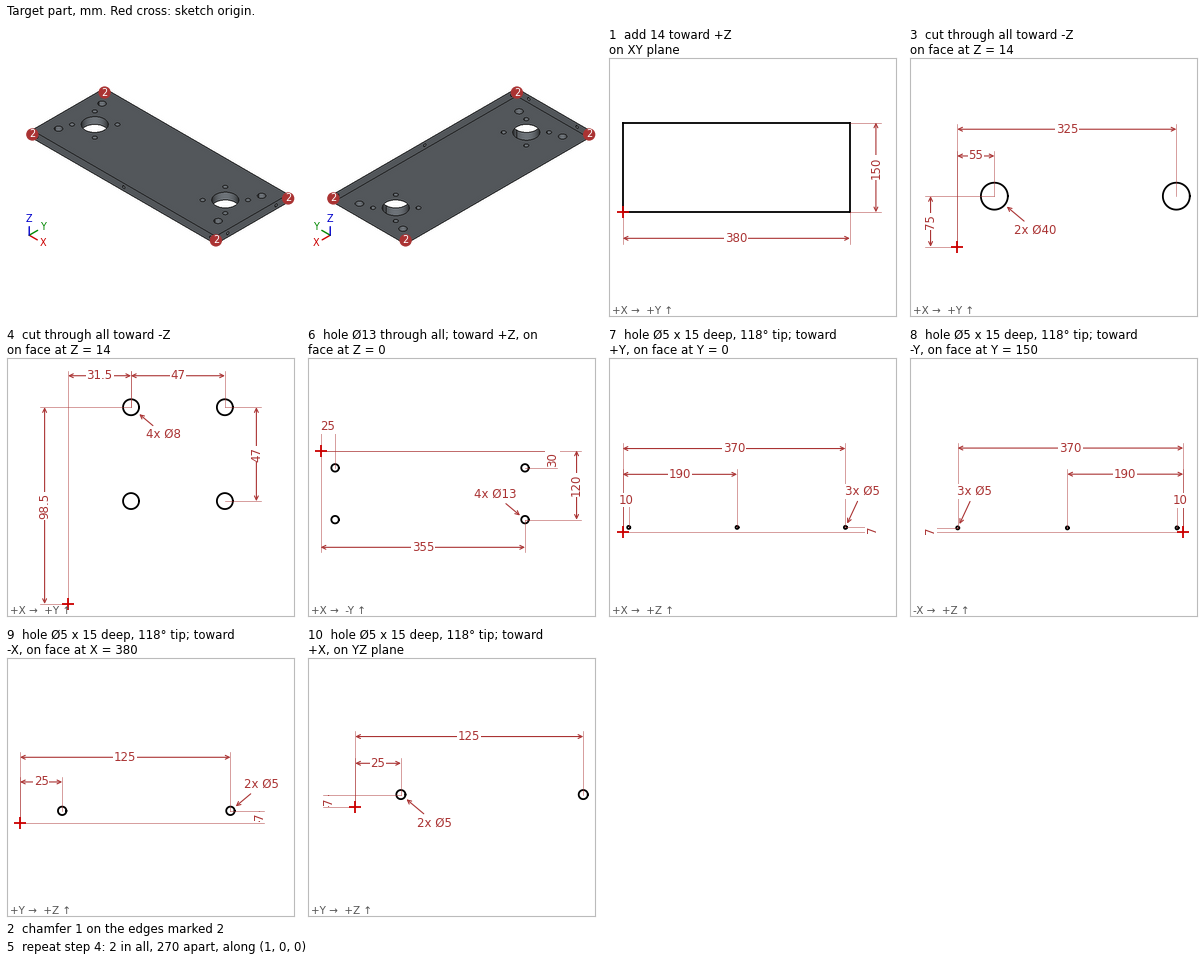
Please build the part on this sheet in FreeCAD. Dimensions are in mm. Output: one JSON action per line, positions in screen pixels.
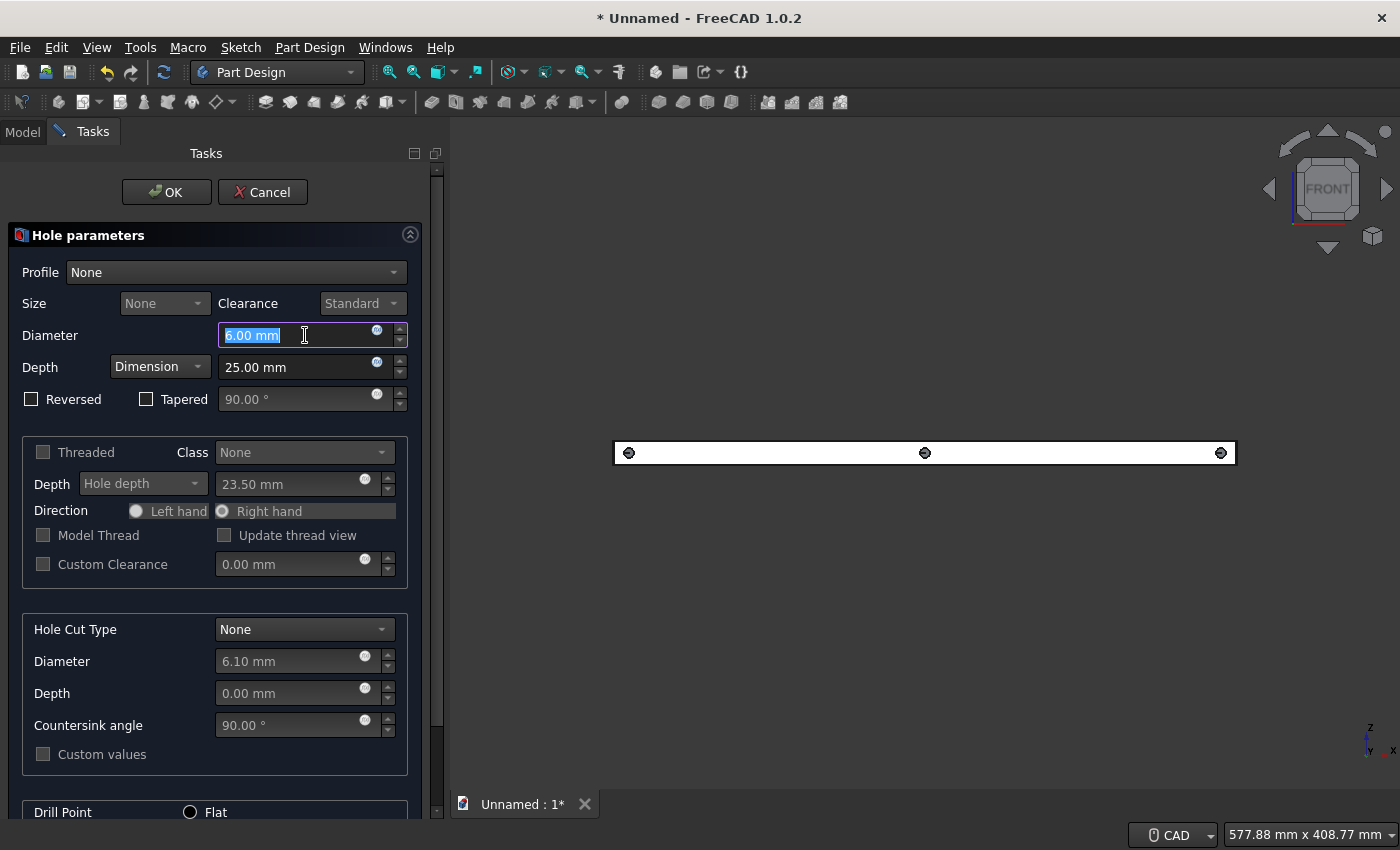
{"action": "type", "text": "5"}
{"action": "key", "text": "Tab"}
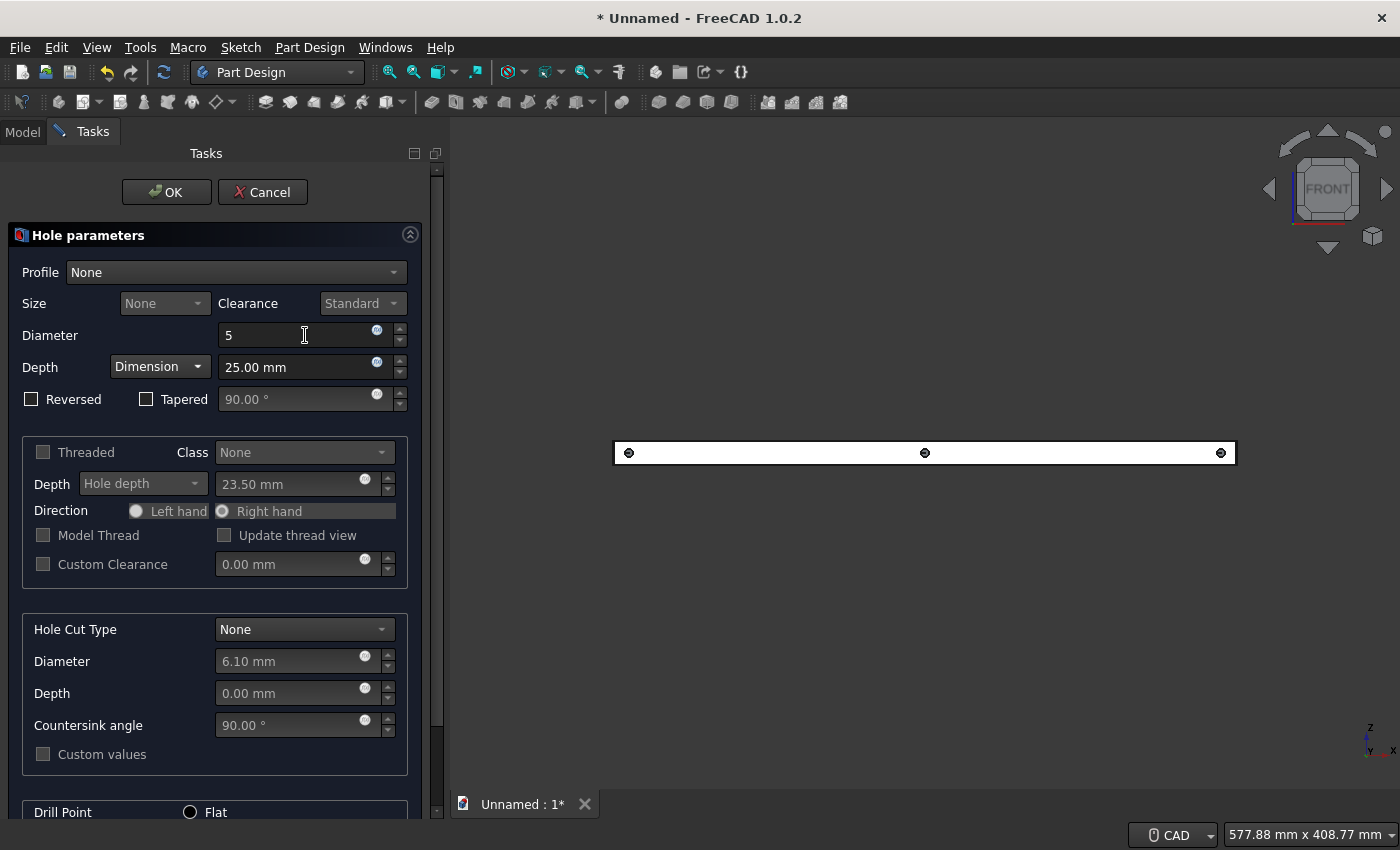
{"action": "triple_click", "coordinate": [305, 367]}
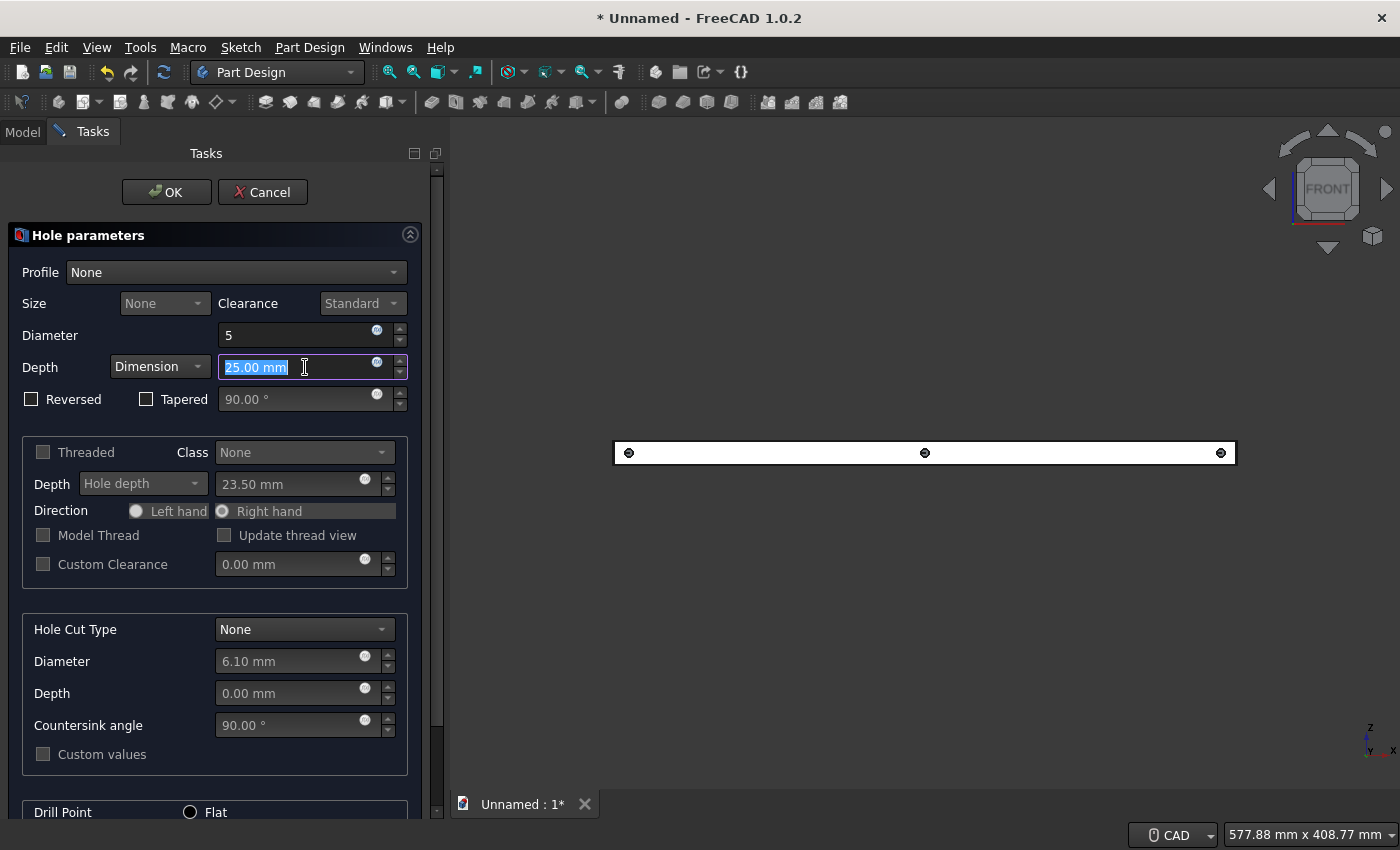
{"action": "type", "text": "15"}
{"action": "key", "text": "Tab"}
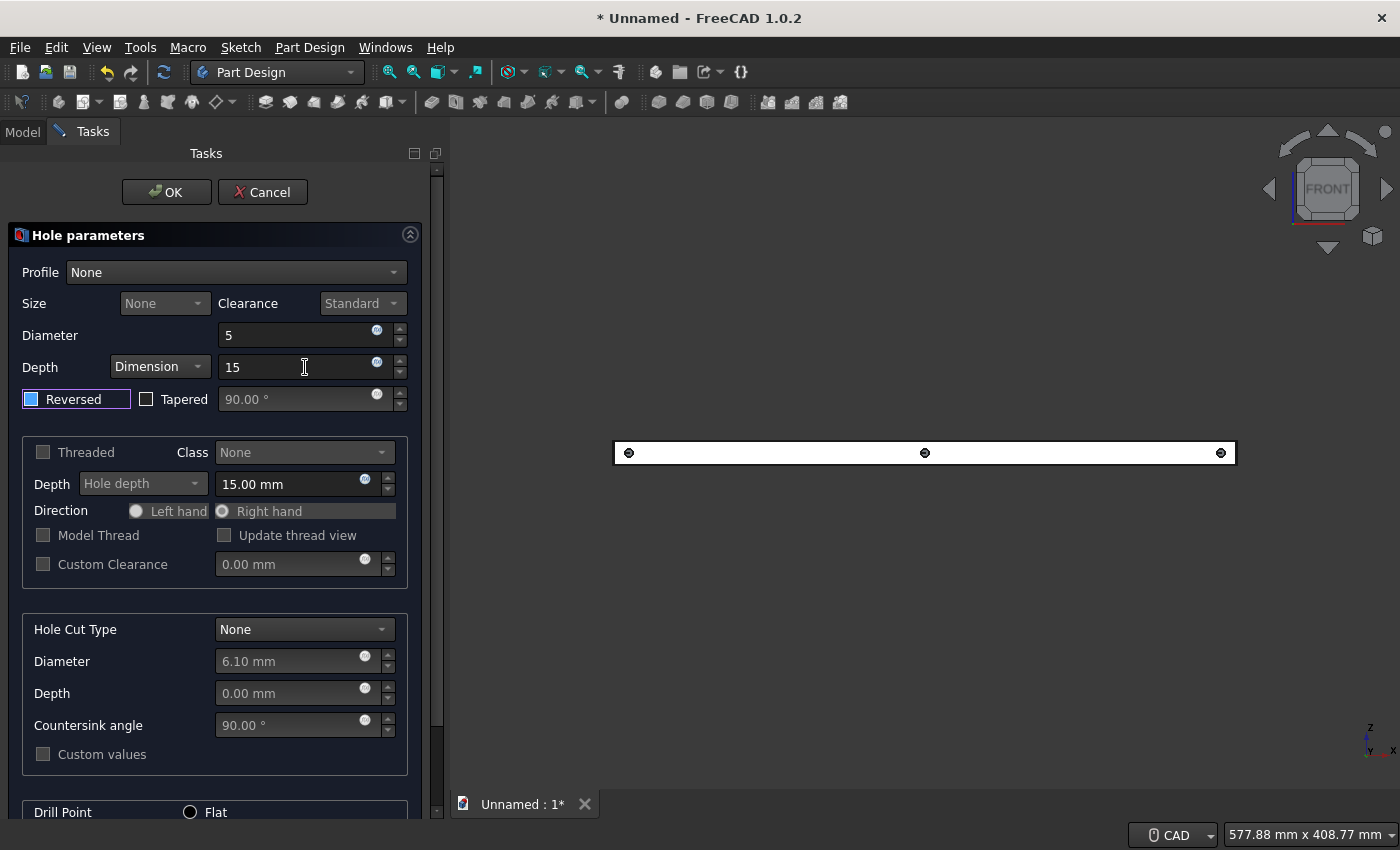
{"action": "left_click", "coordinate": [167, 192]}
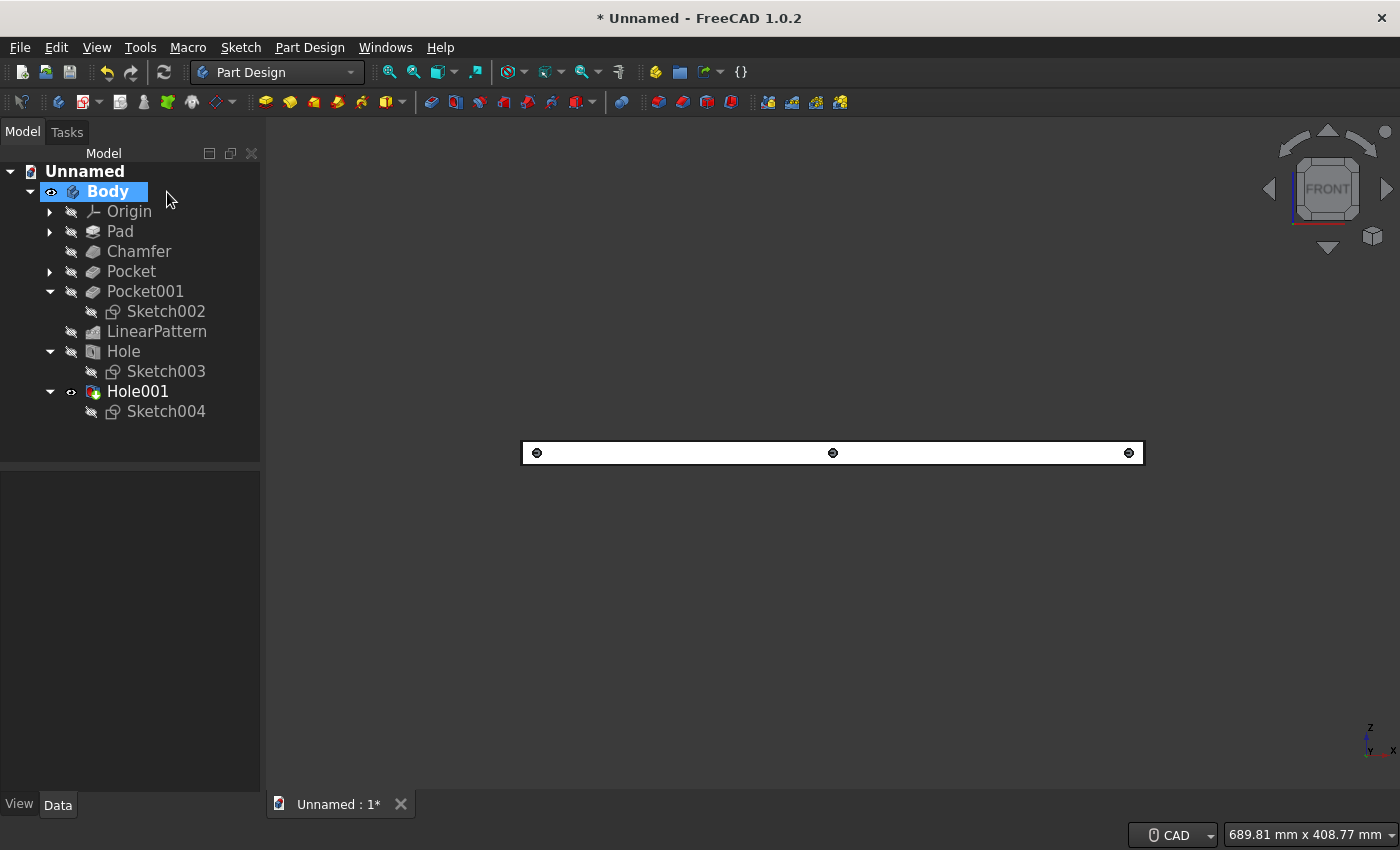
{"action": "key", "text": "4"}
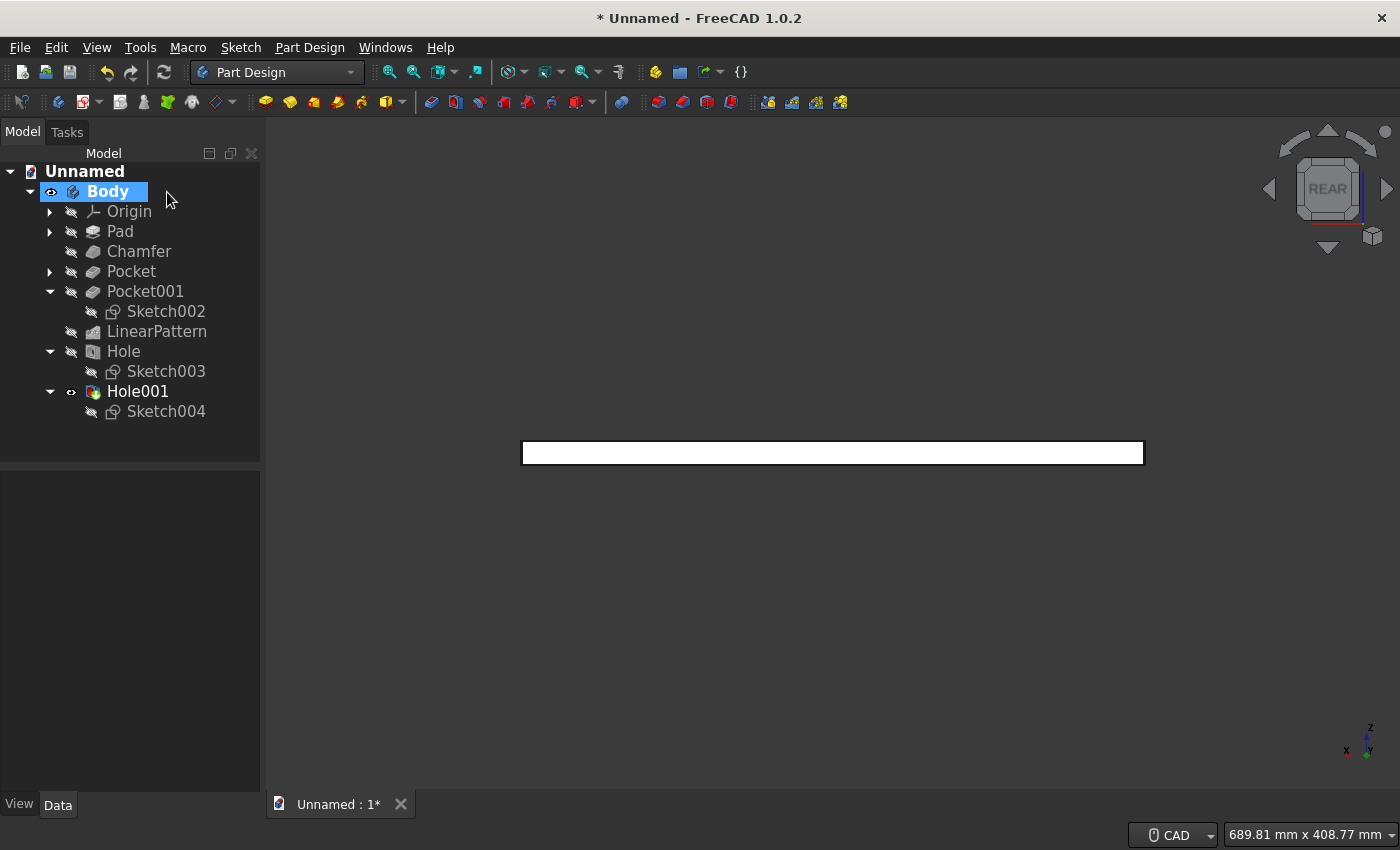
{"action": "left_click", "coordinate": [567, 452]}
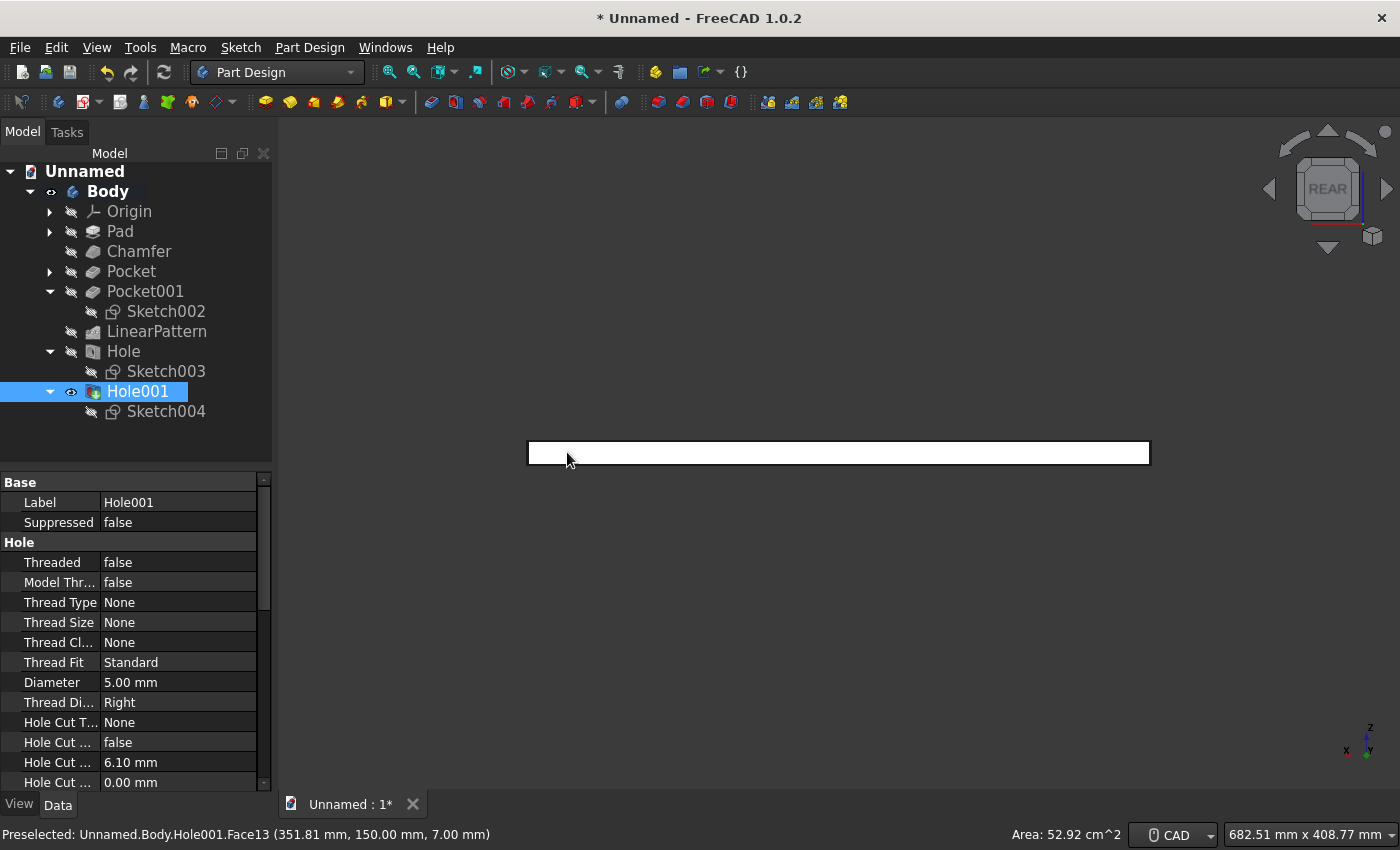
{"action": "left_click", "coordinate": [84, 102]}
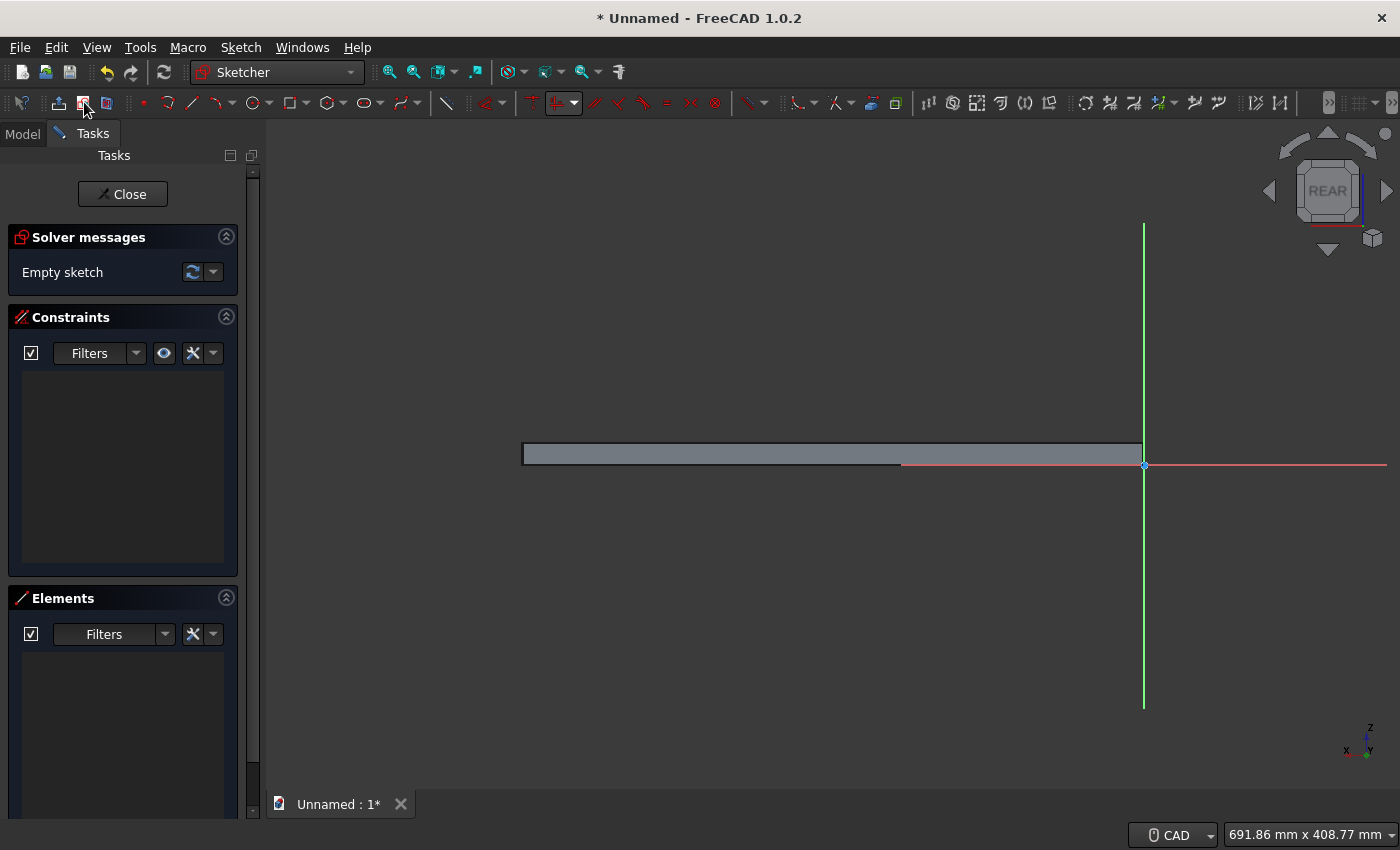
{"action": "left_click", "coordinate": [254, 104]}